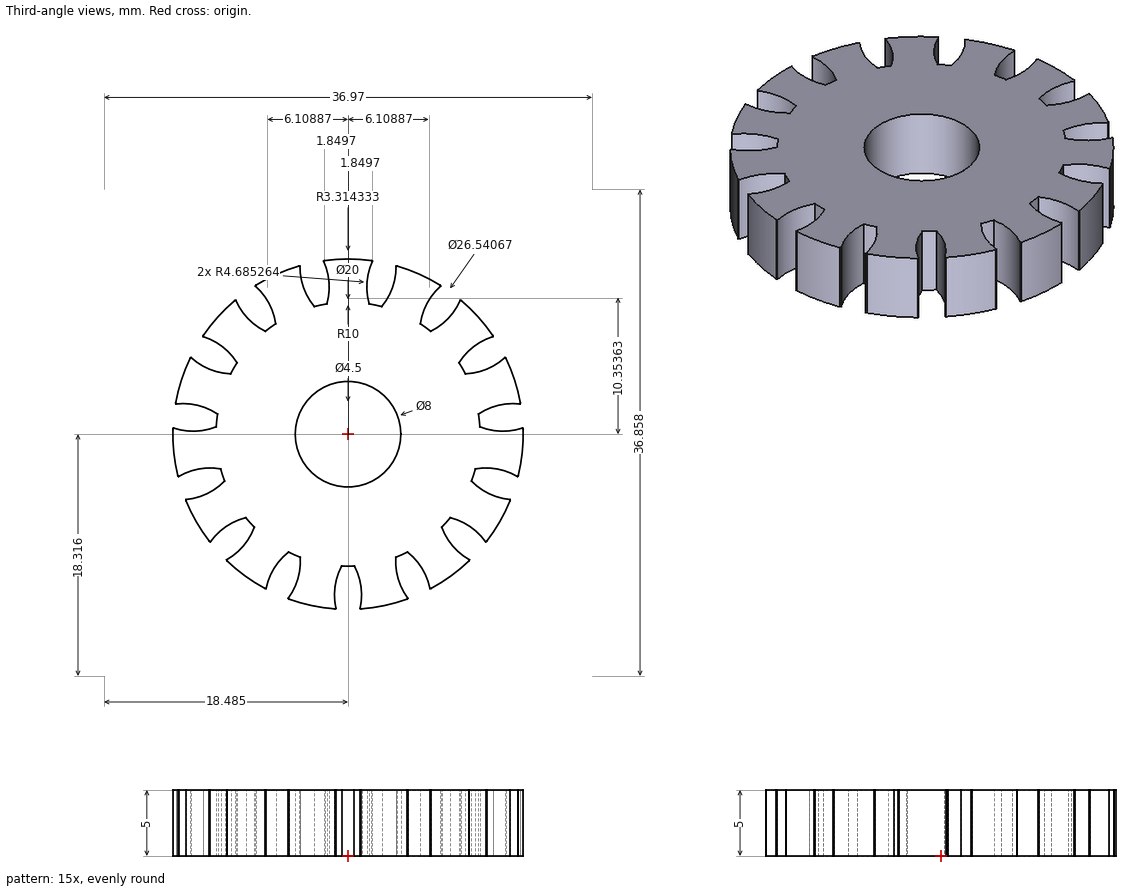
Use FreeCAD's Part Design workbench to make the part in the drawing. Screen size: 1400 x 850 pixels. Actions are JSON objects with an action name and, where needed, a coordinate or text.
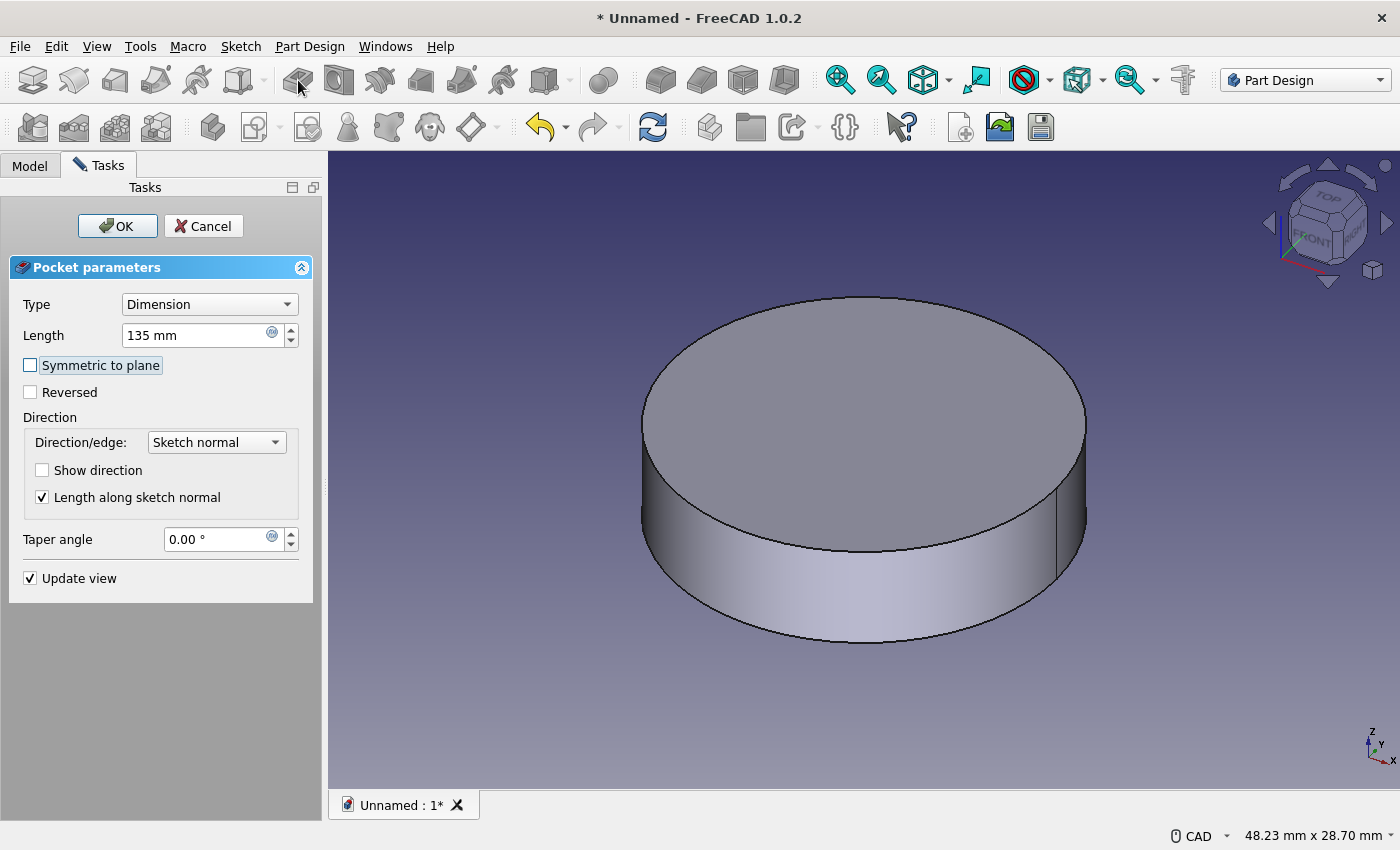
{"action": "left_click", "coordinate": [31, 365]}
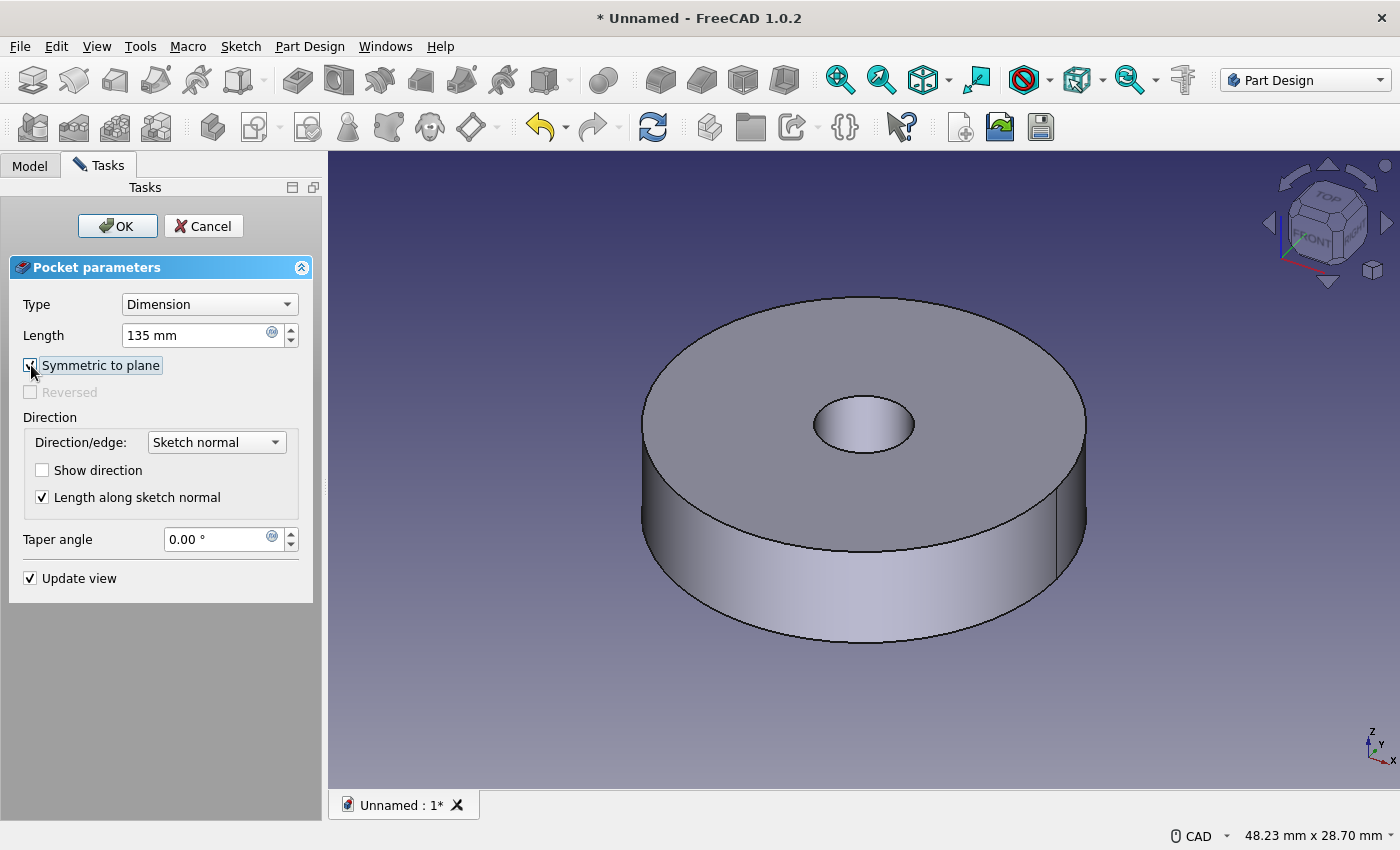
{"action": "left_click", "coordinate": [118, 226]}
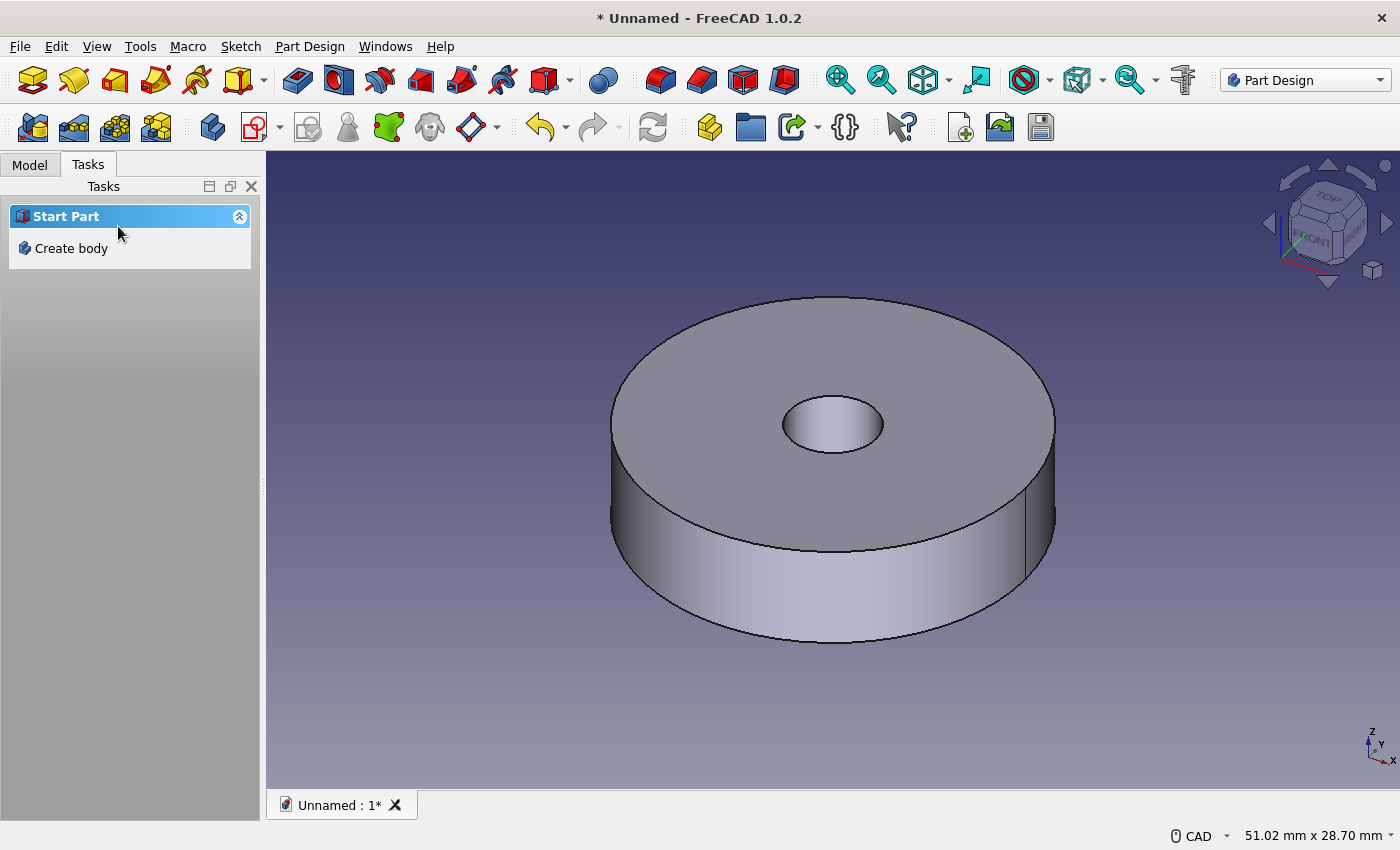
{"action": "left_click", "coordinate": [254, 128]}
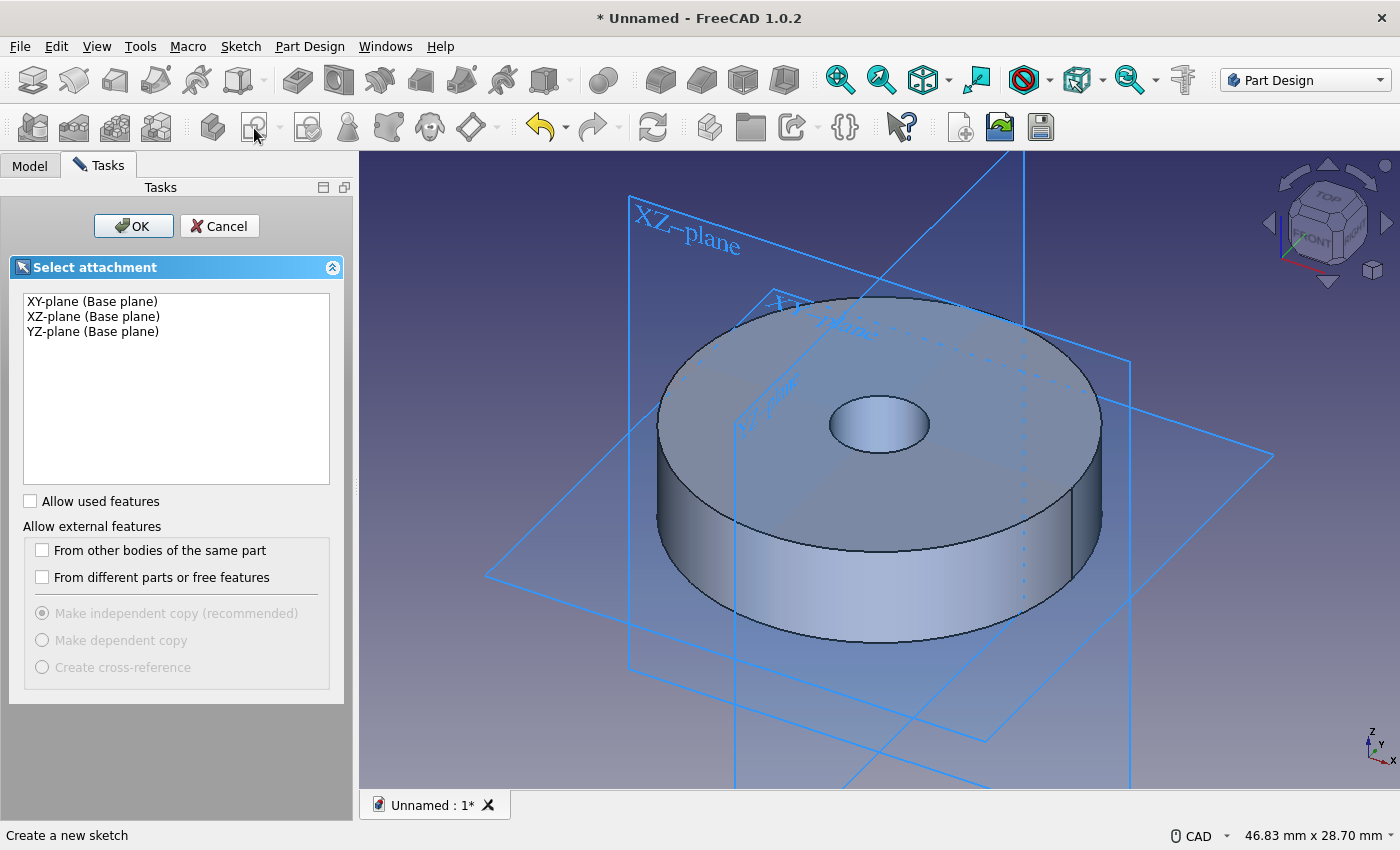
{"action": "left_click", "coordinate": [84, 302]}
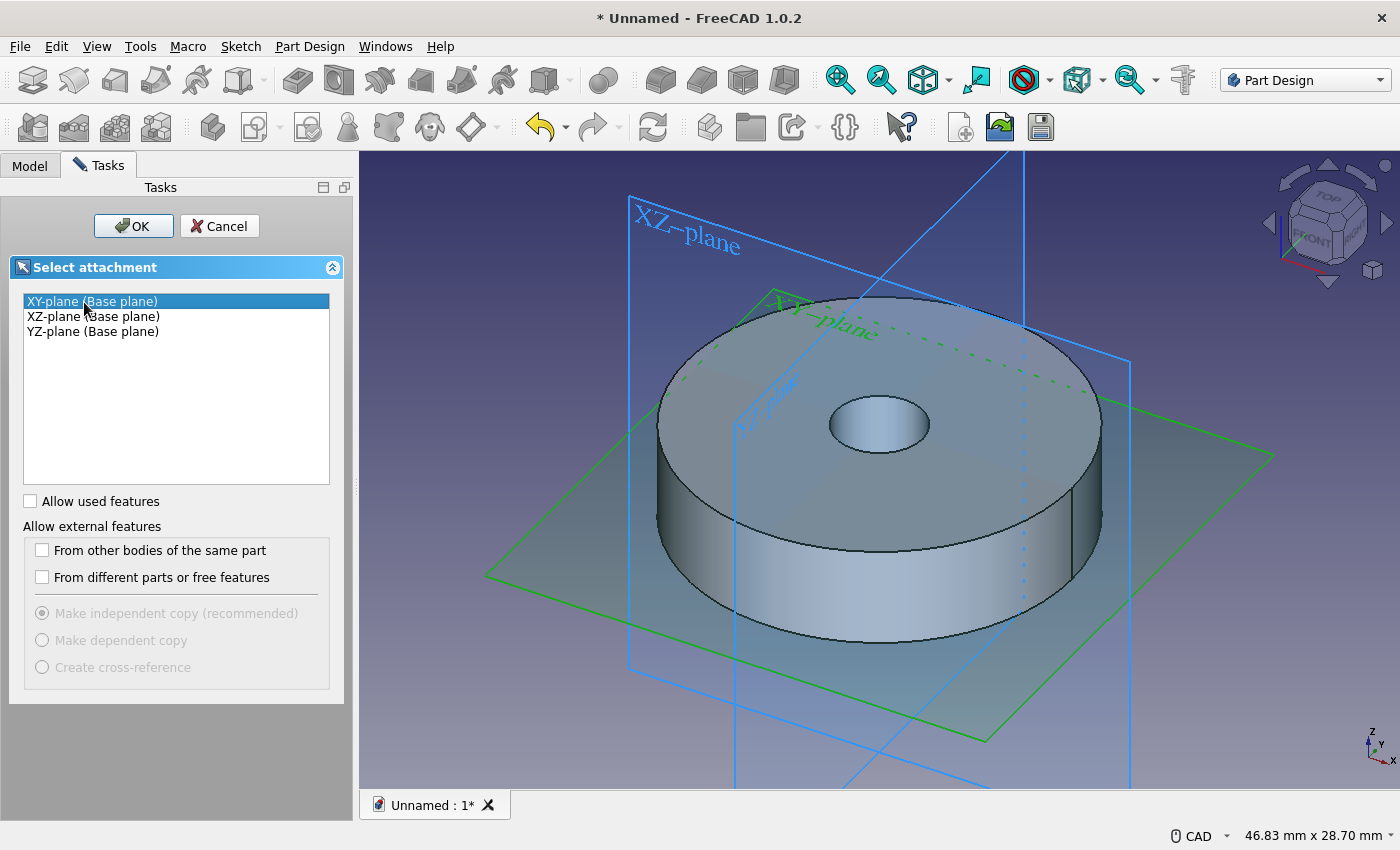
{"action": "left_click", "coordinate": [134, 226]}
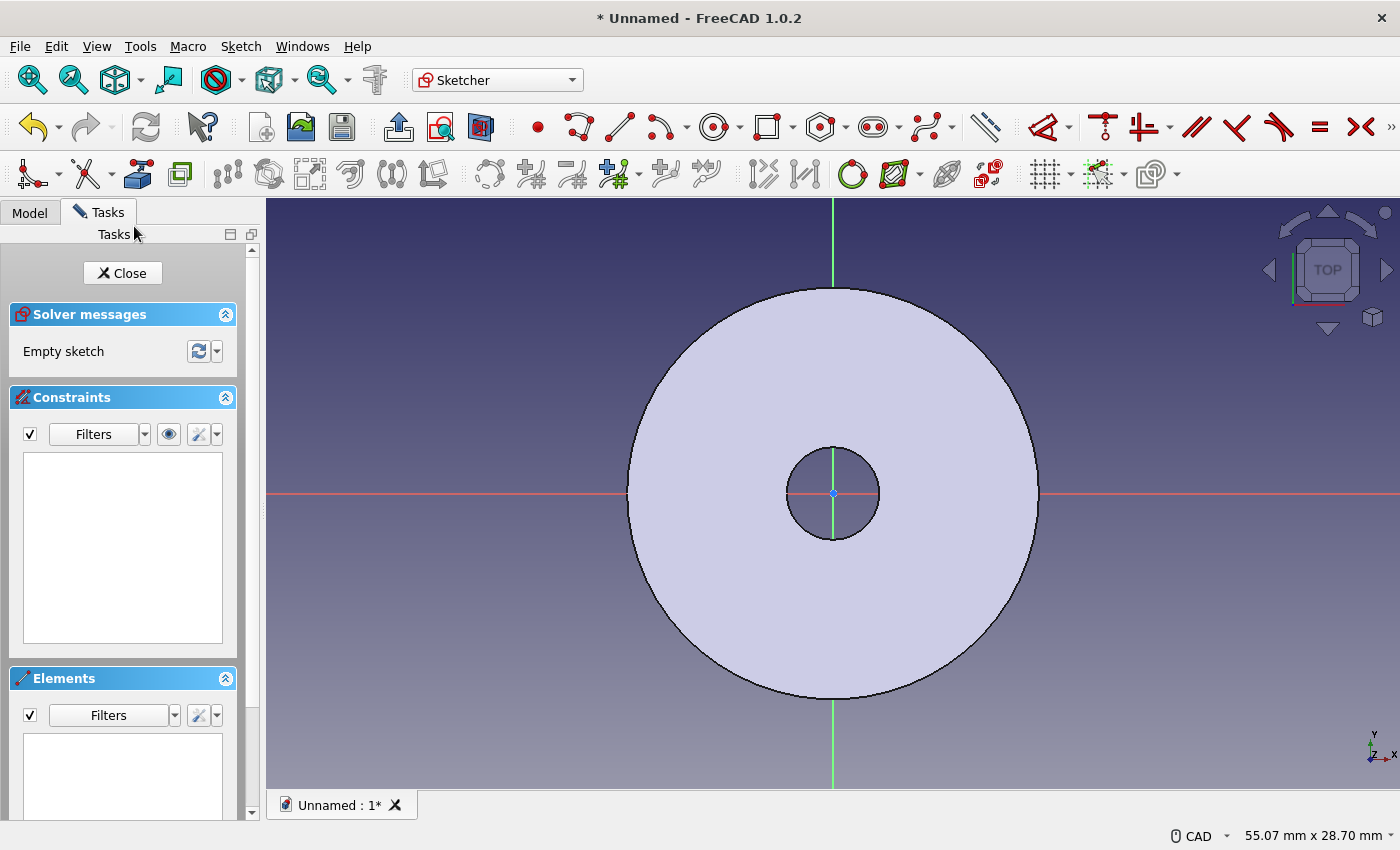
{"action": "left_click", "coordinate": [481, 128]}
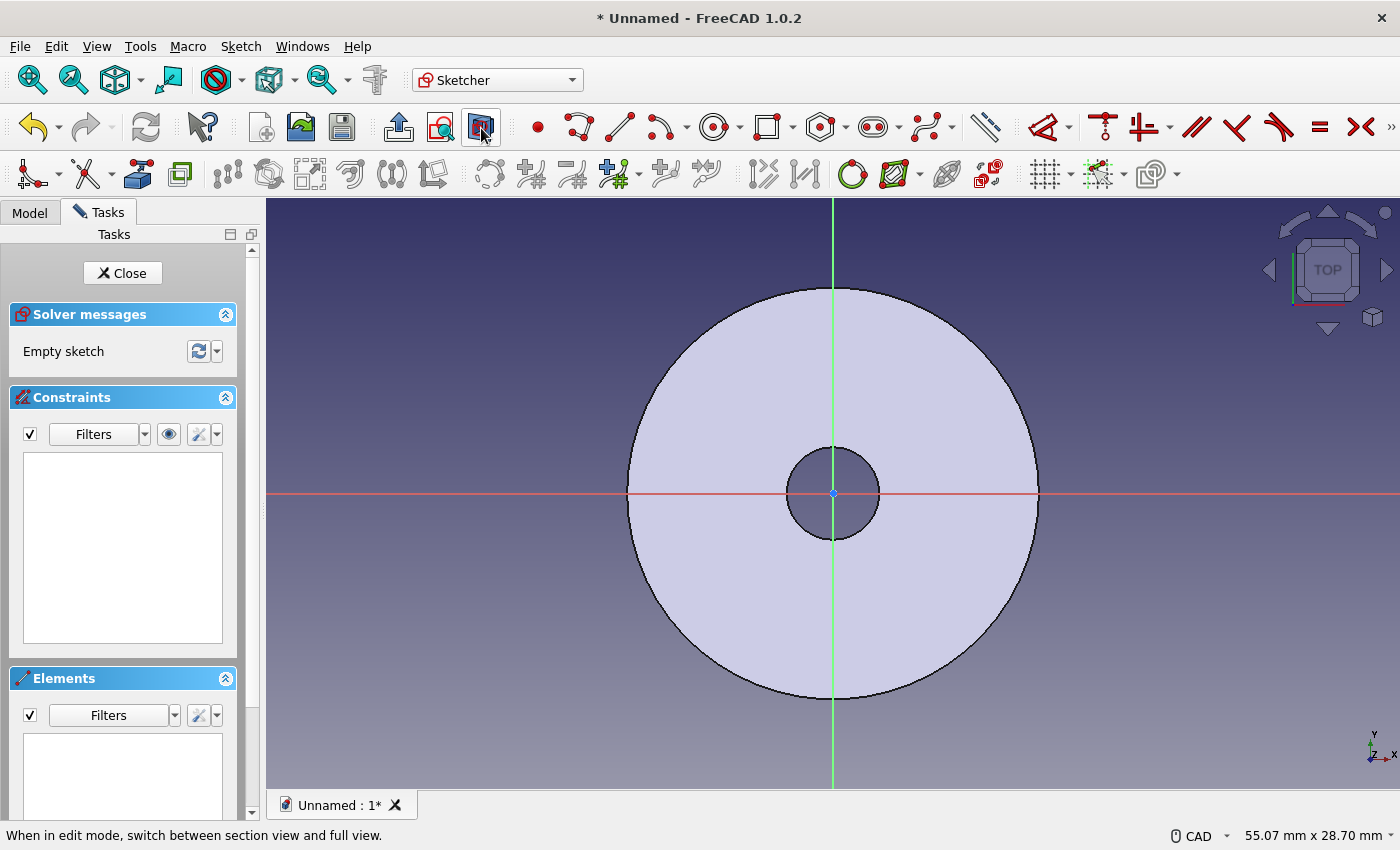
{"action": "scroll", "coordinate": [764, 494], "scroll_direction": "down", "scroll_amount": 5}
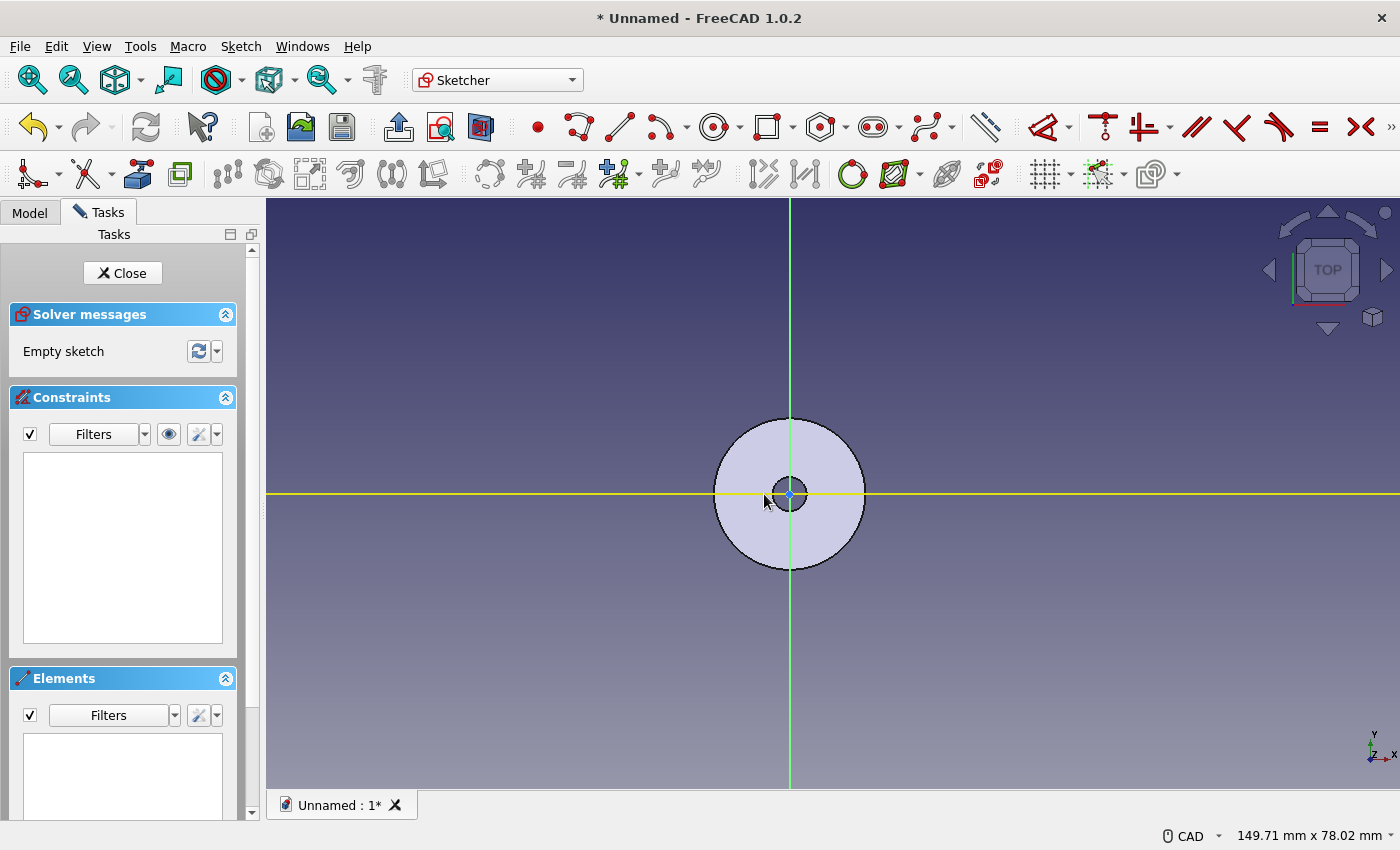
{"action": "scroll", "coordinate": [792, 398], "scroll_direction": "up", "scroll_amount": 13}